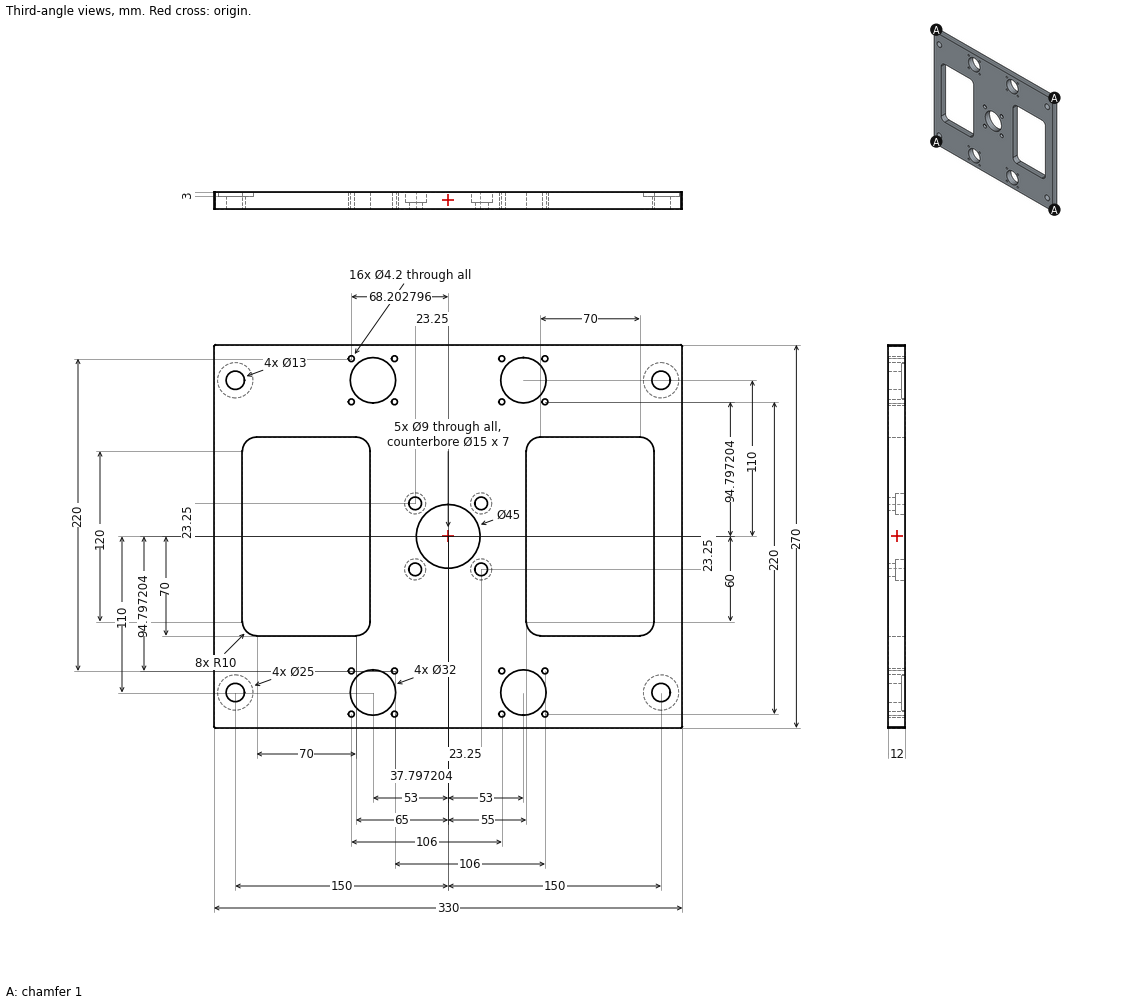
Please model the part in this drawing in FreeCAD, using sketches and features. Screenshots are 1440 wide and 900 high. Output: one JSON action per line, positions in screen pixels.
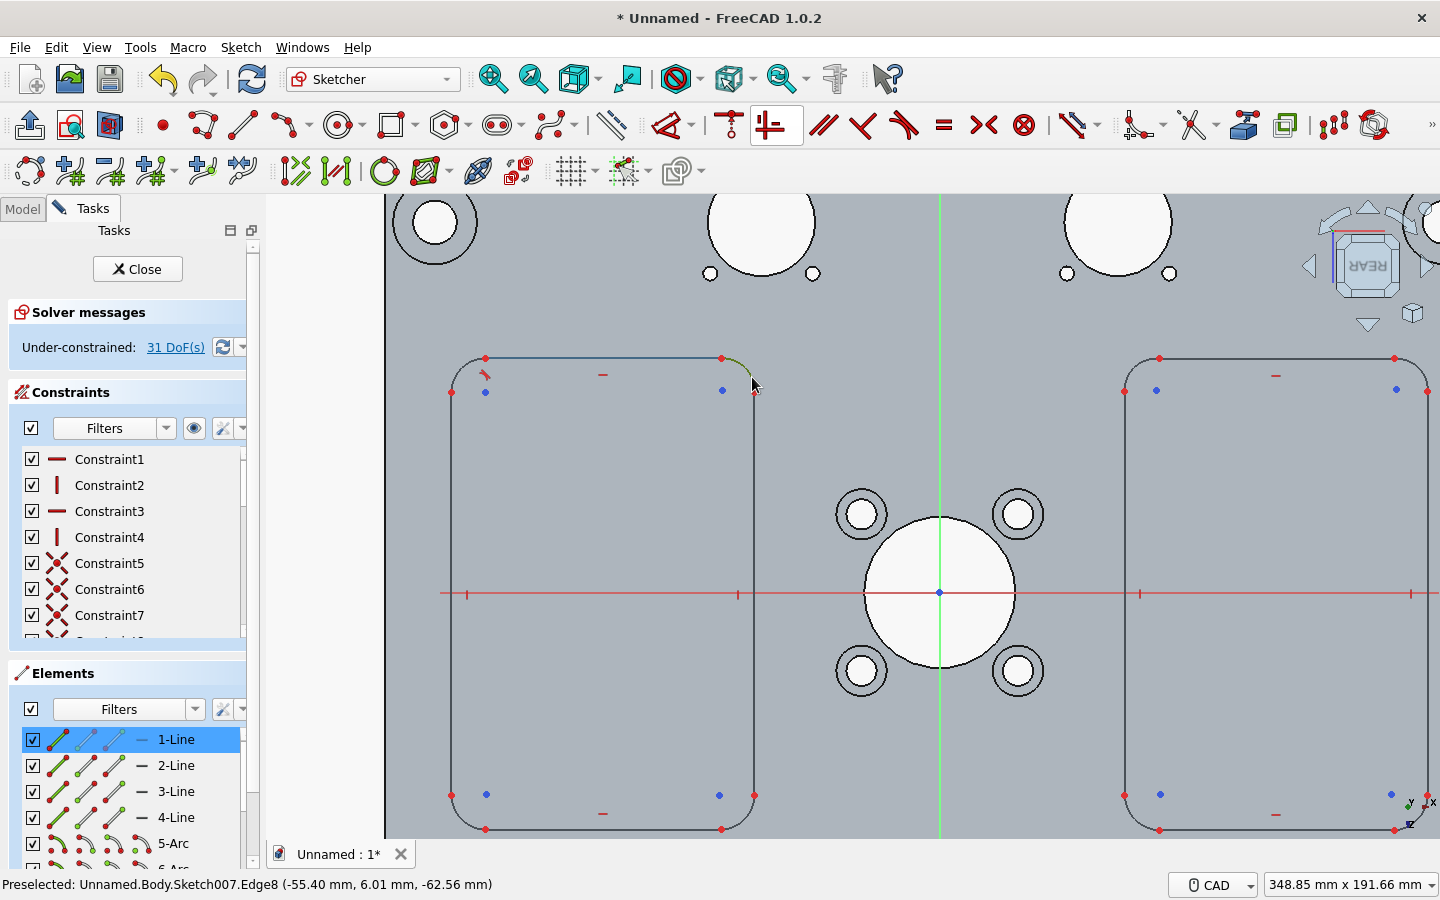
{"action": "left_click", "coordinate": [904, 126]}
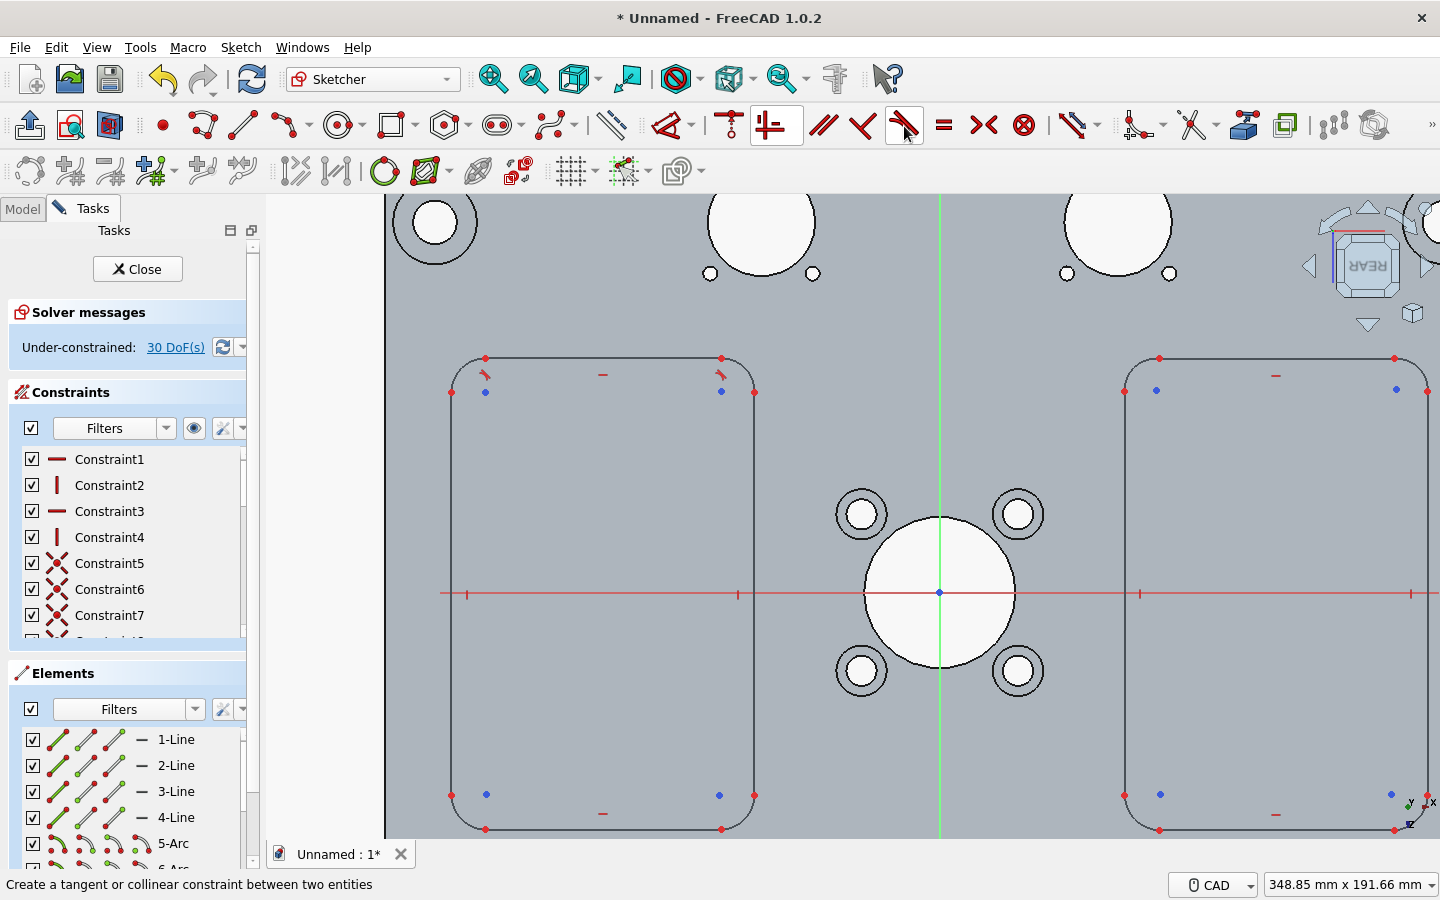
{"action": "left_click", "coordinate": [451, 513]}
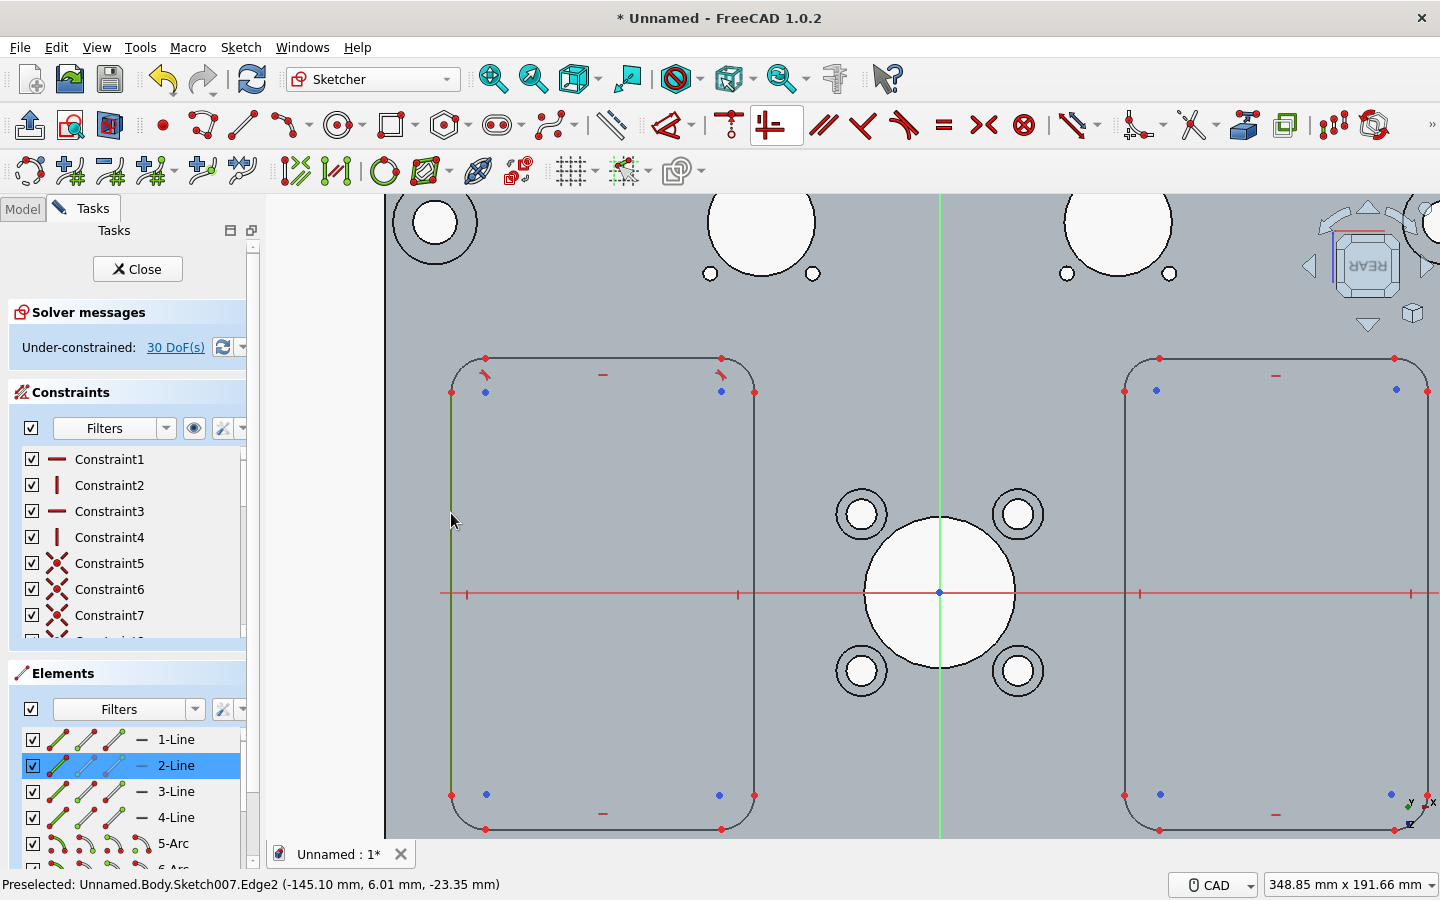
{"action": "left_click", "coordinate": [470, 362]}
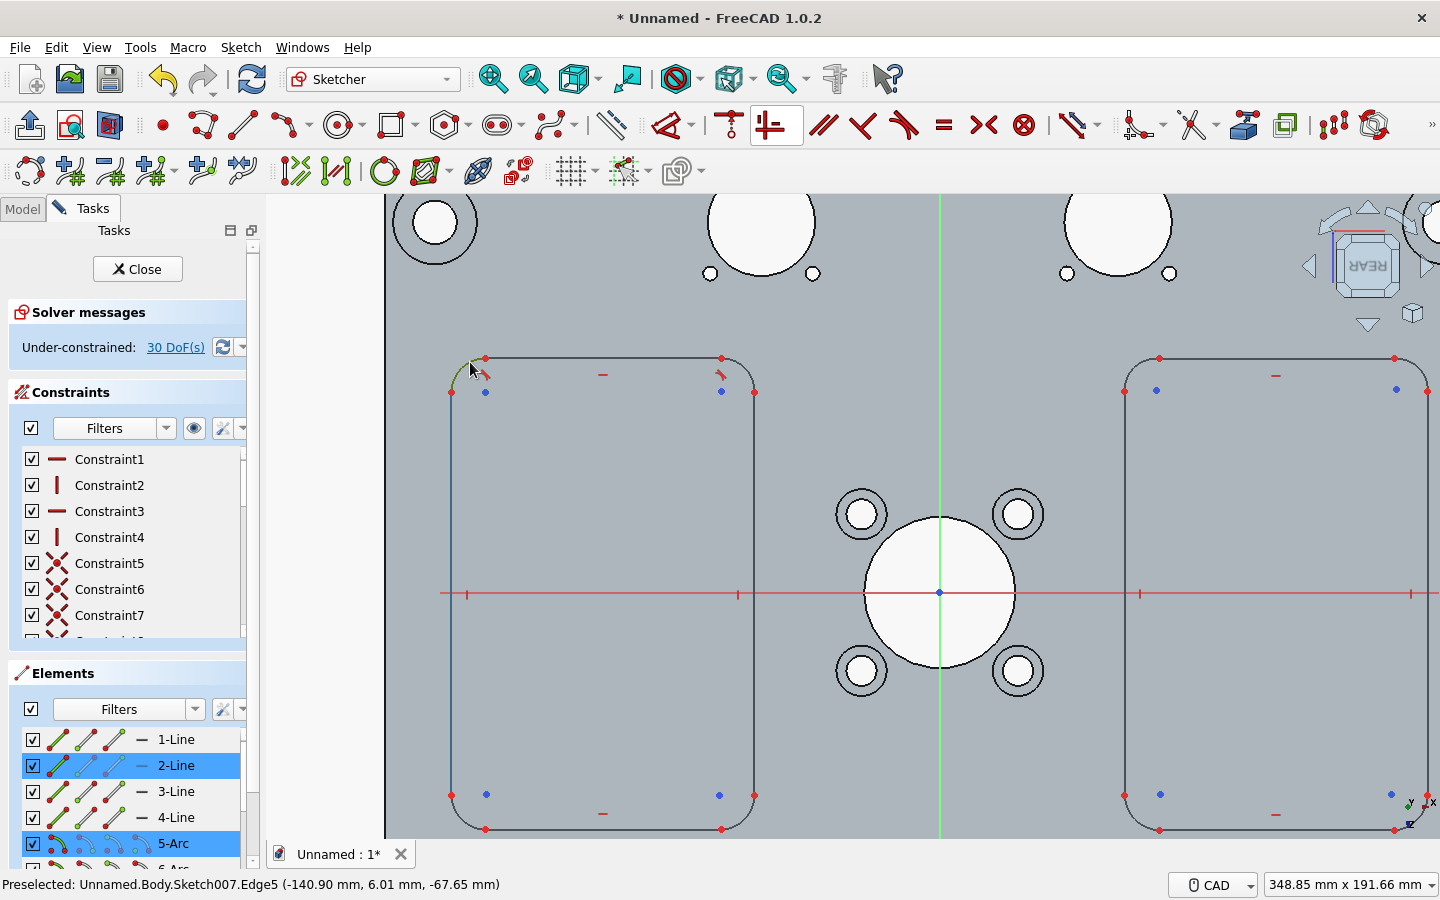
{"action": "left_click", "coordinate": [904, 126]}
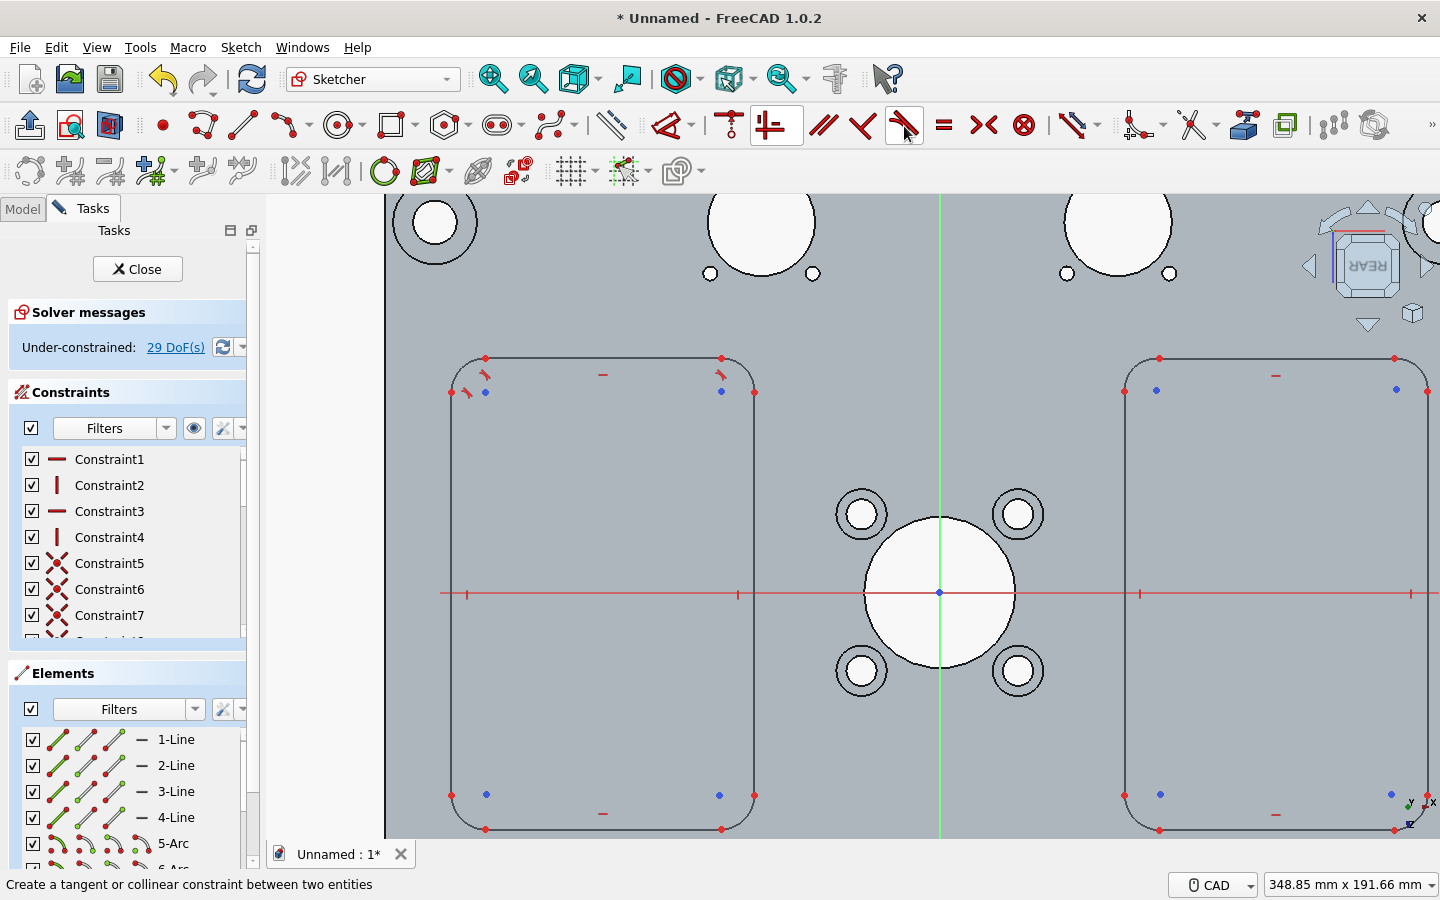
{"action": "left_click", "coordinate": [451, 513]}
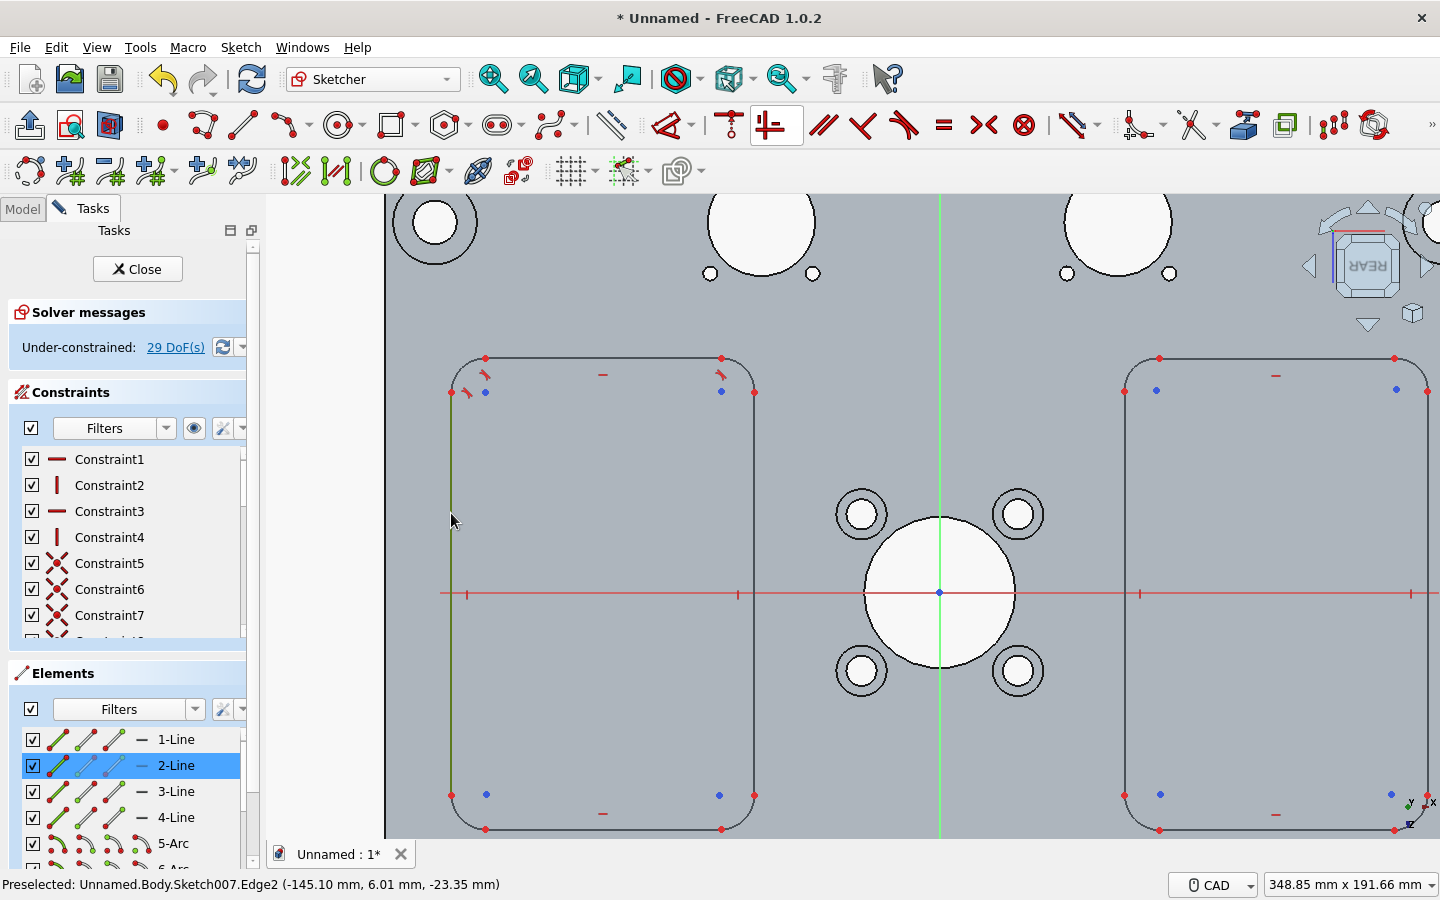
{"action": "left_click", "coordinate": [456, 811]}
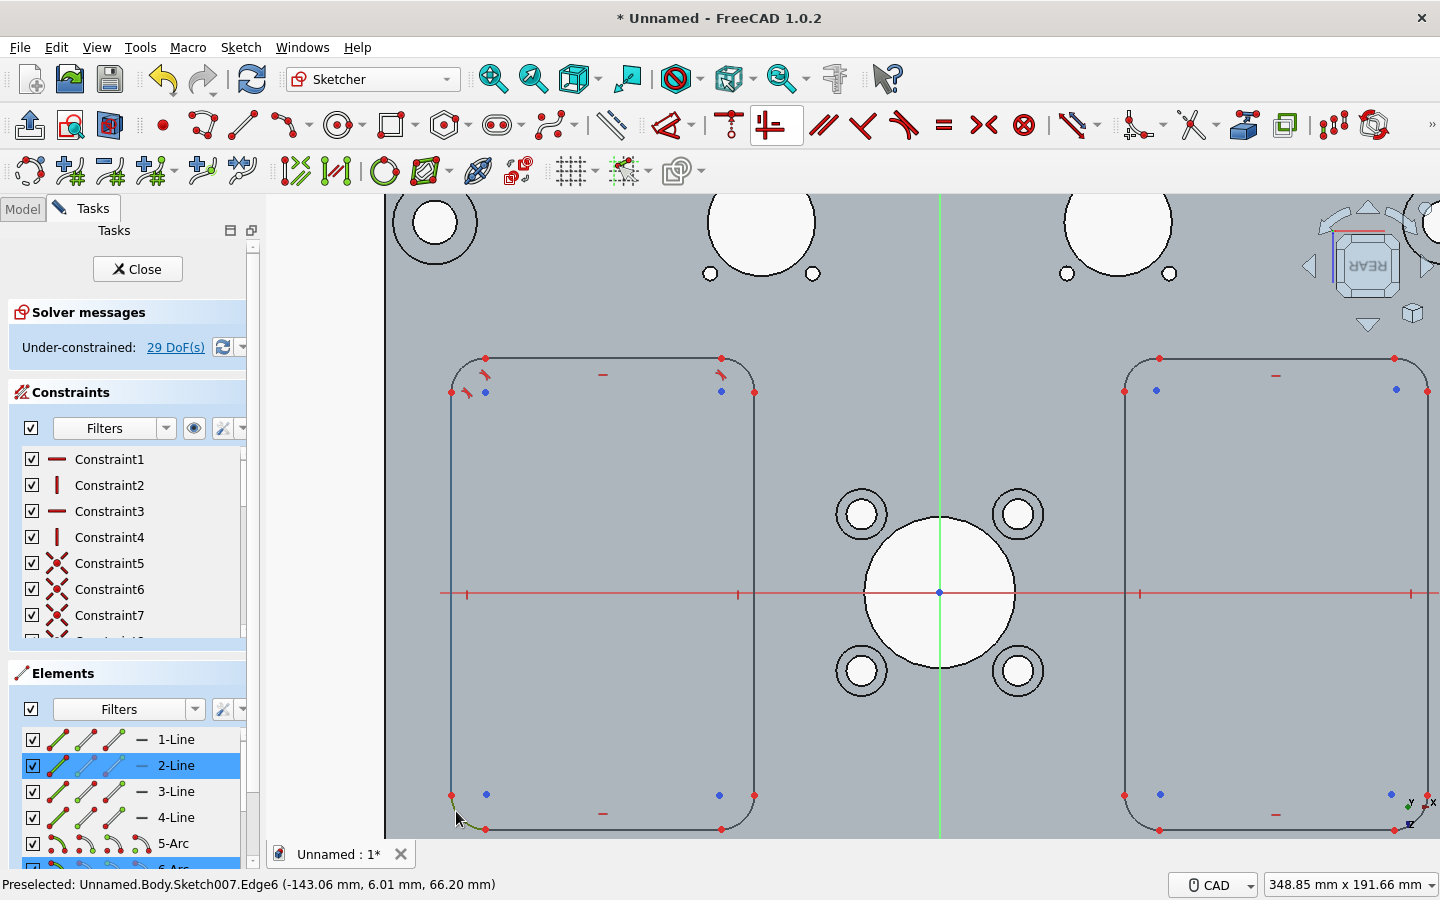
{"action": "left_click", "coordinate": [904, 126]}